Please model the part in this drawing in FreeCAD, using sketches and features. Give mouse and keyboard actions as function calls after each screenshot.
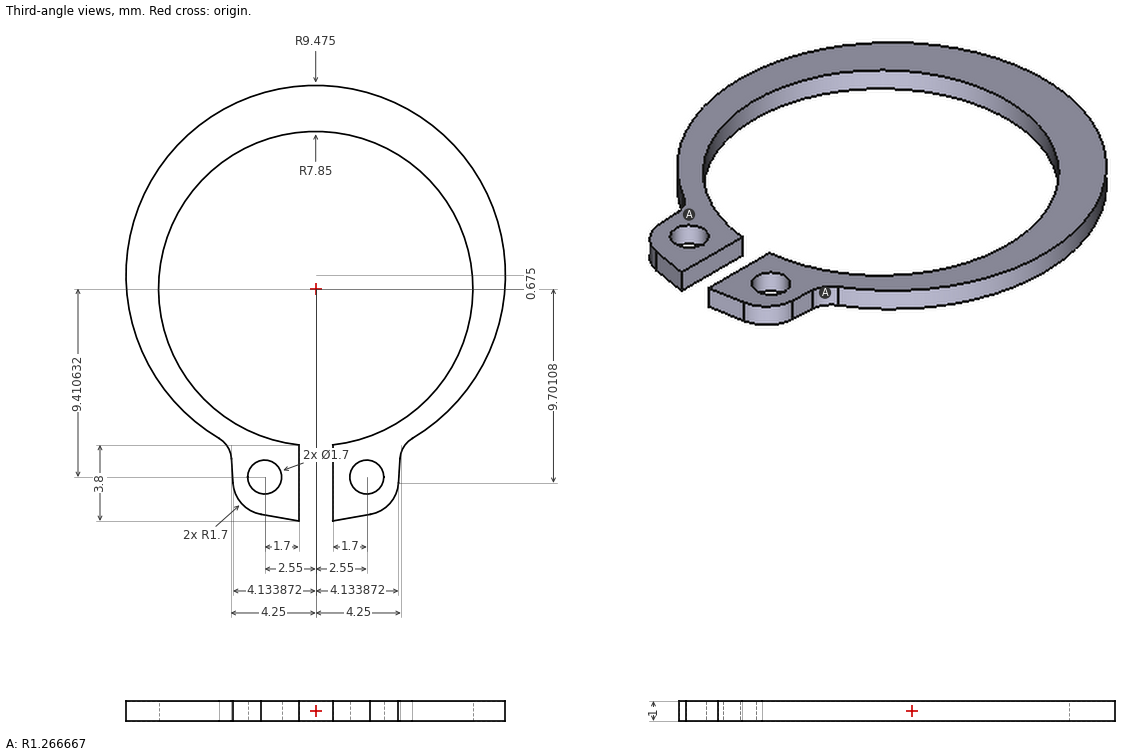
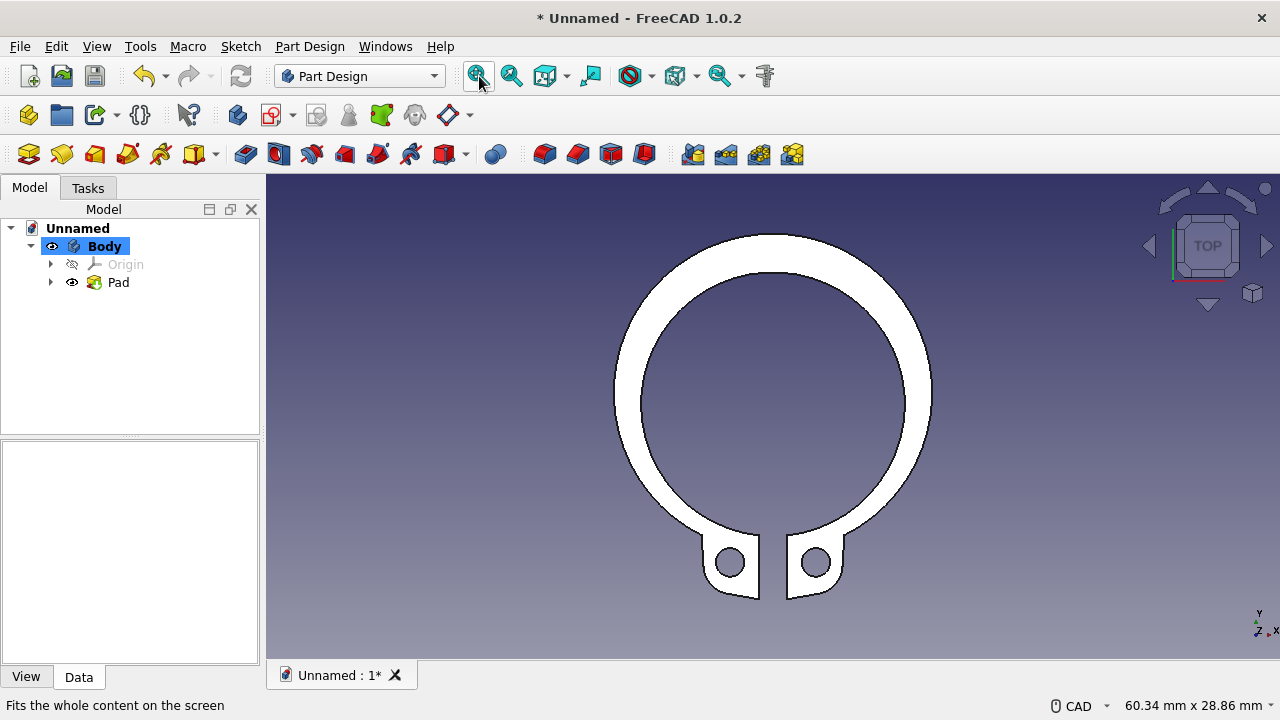
key(1)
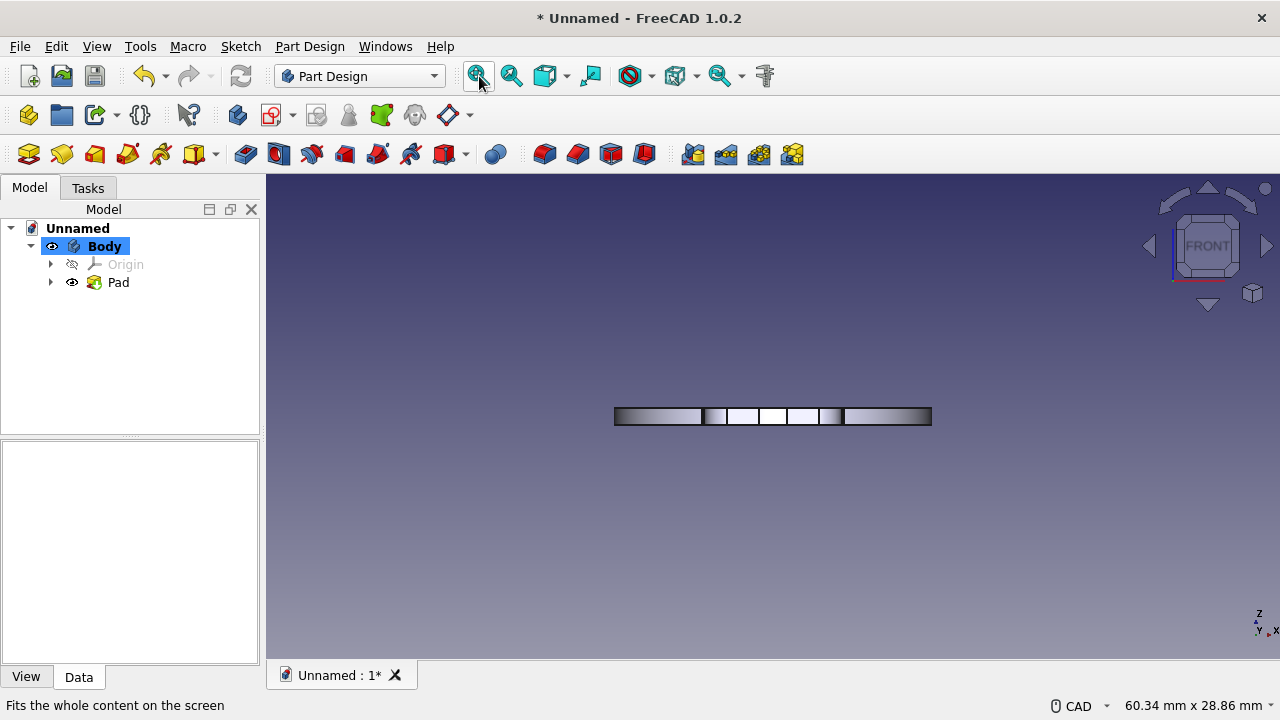
click(479, 76)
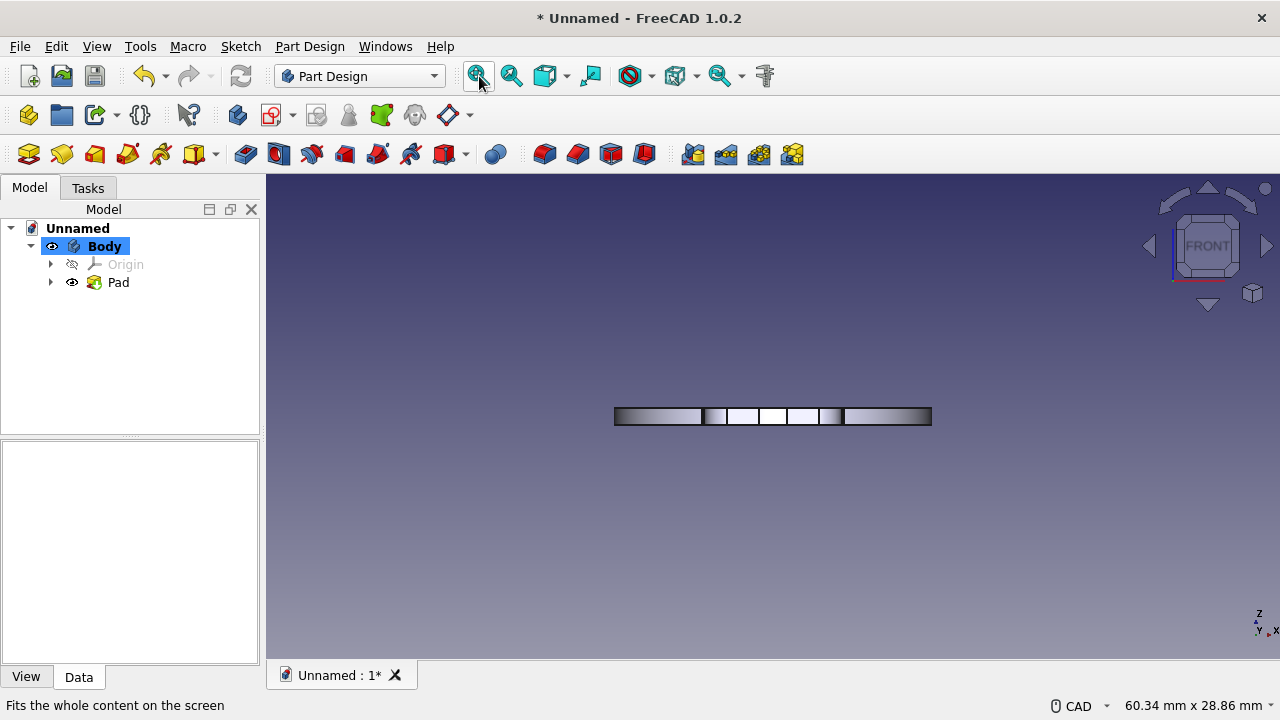
scroll(702, 416, up, 5)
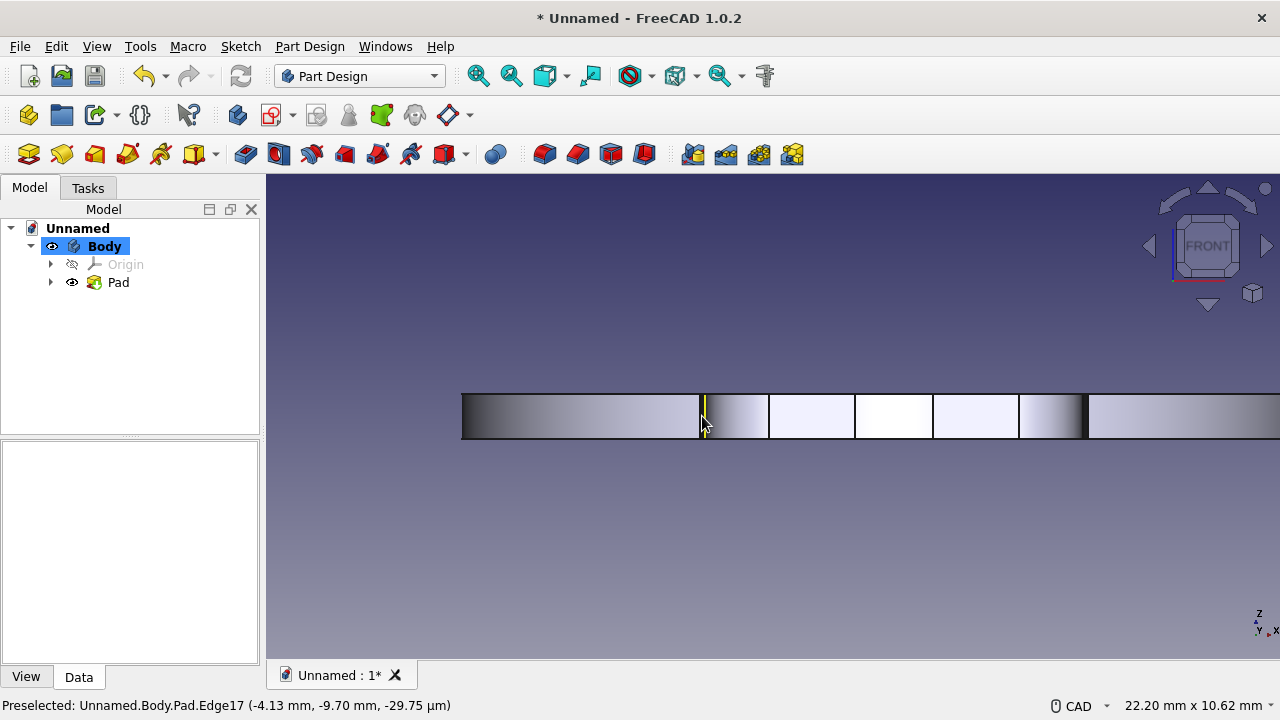
click(479, 76)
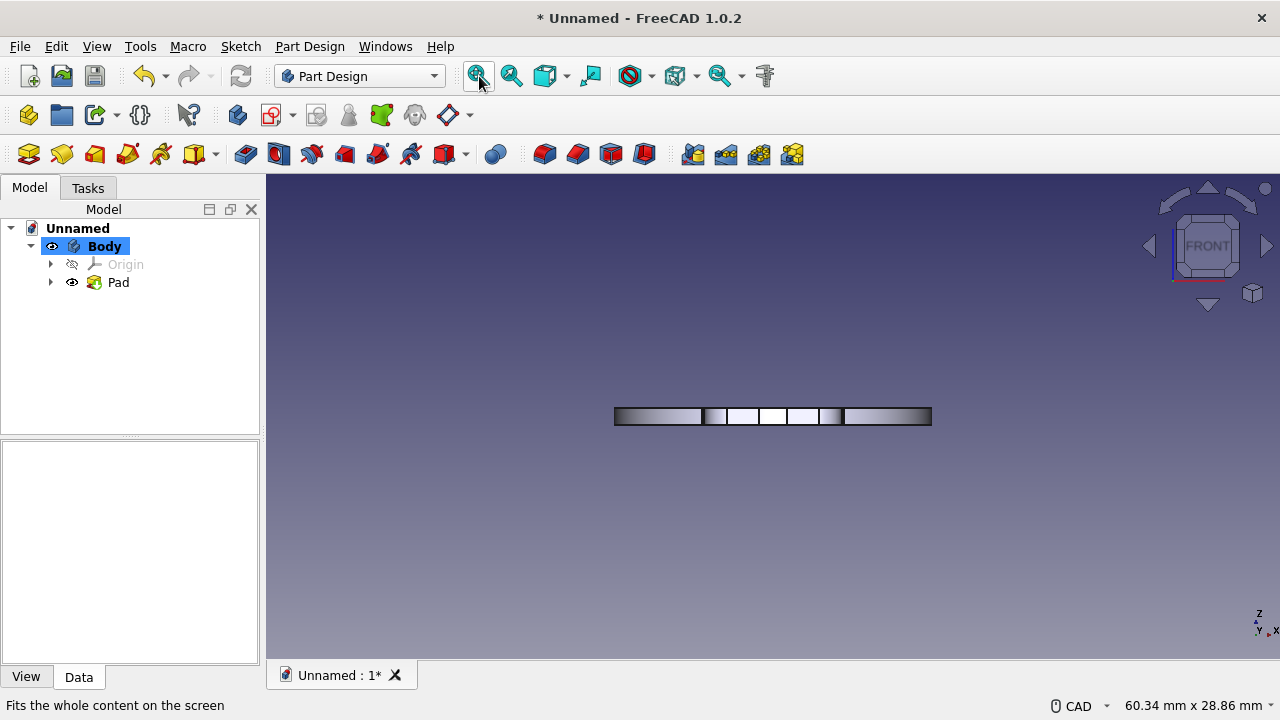
key(3)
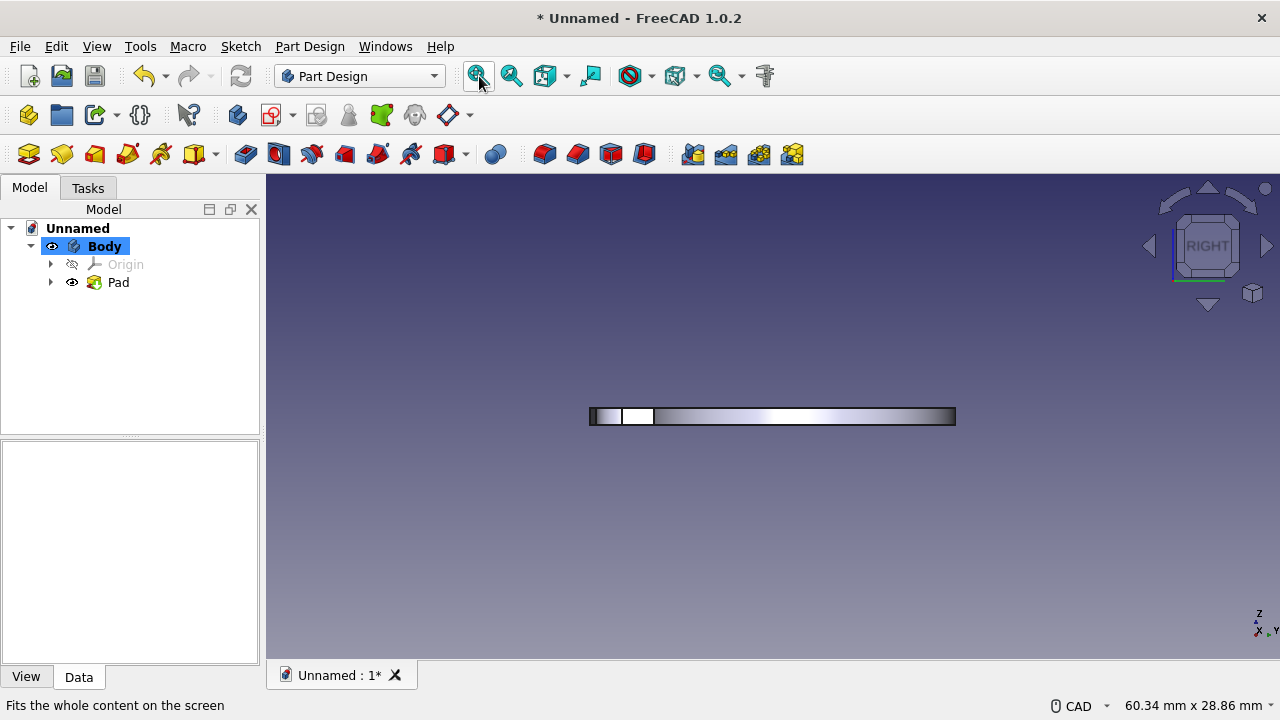
click(479, 76)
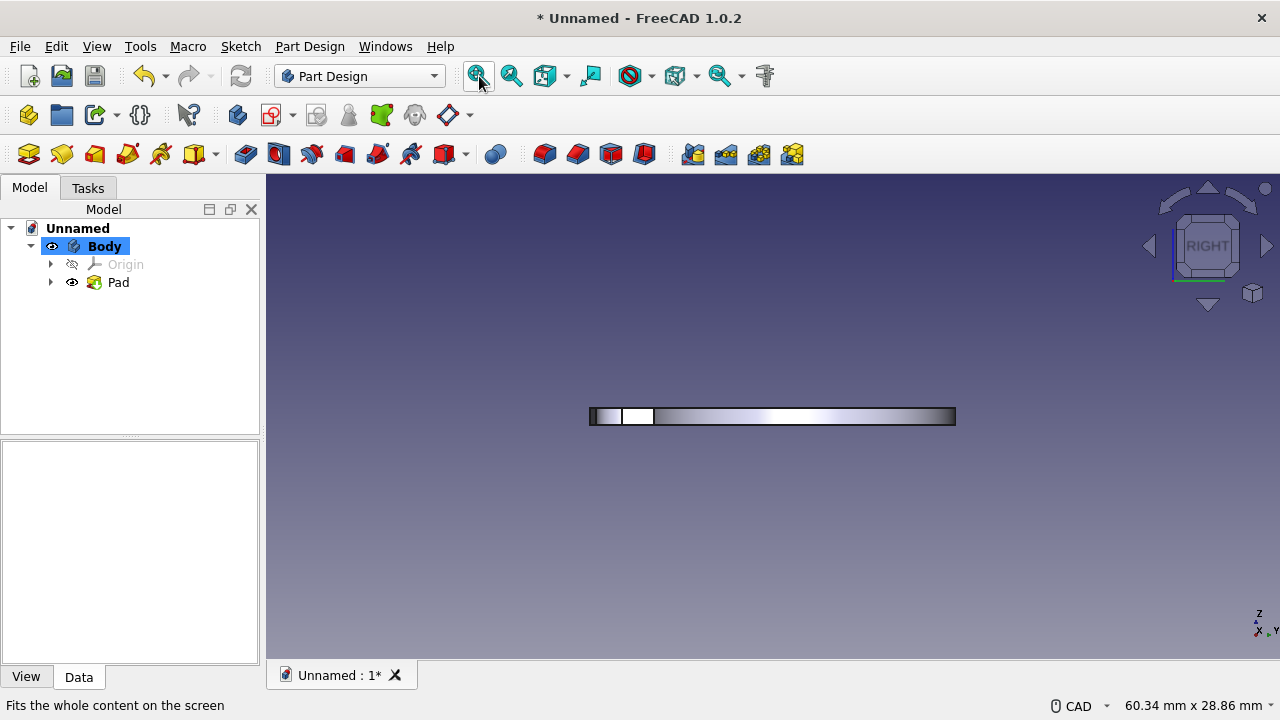
scroll(654, 415, up, 5)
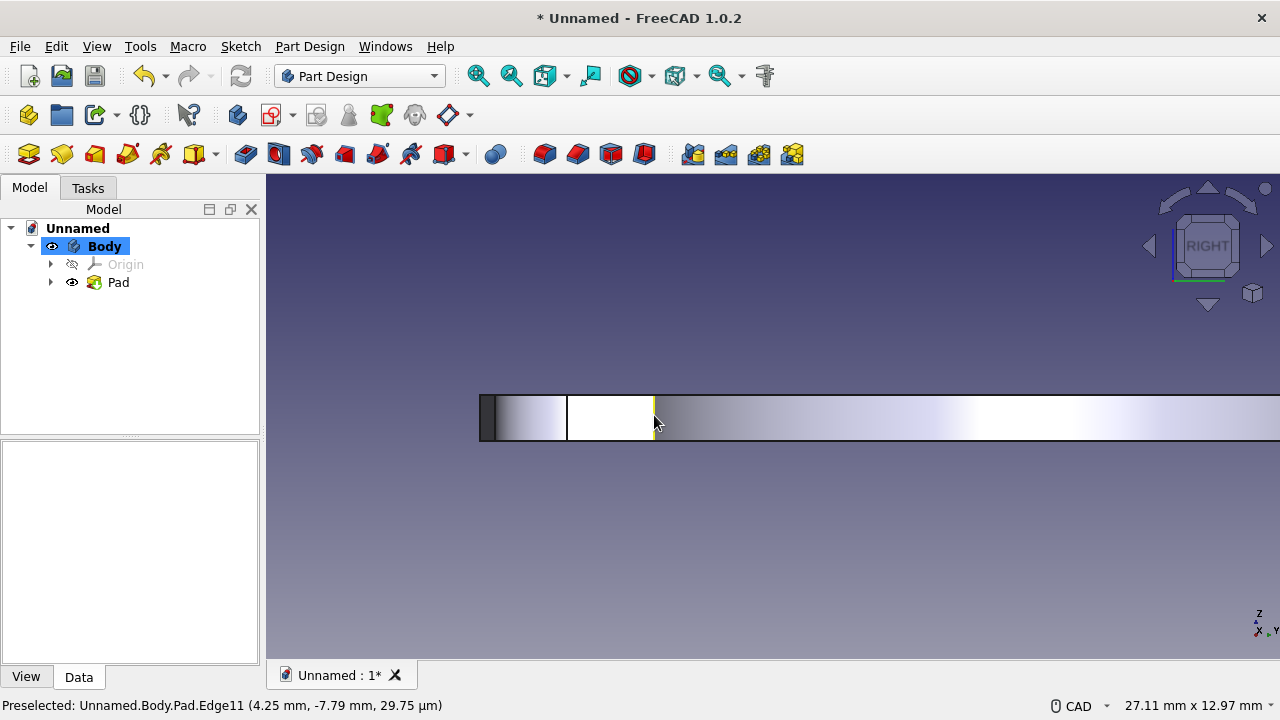
click(479, 76)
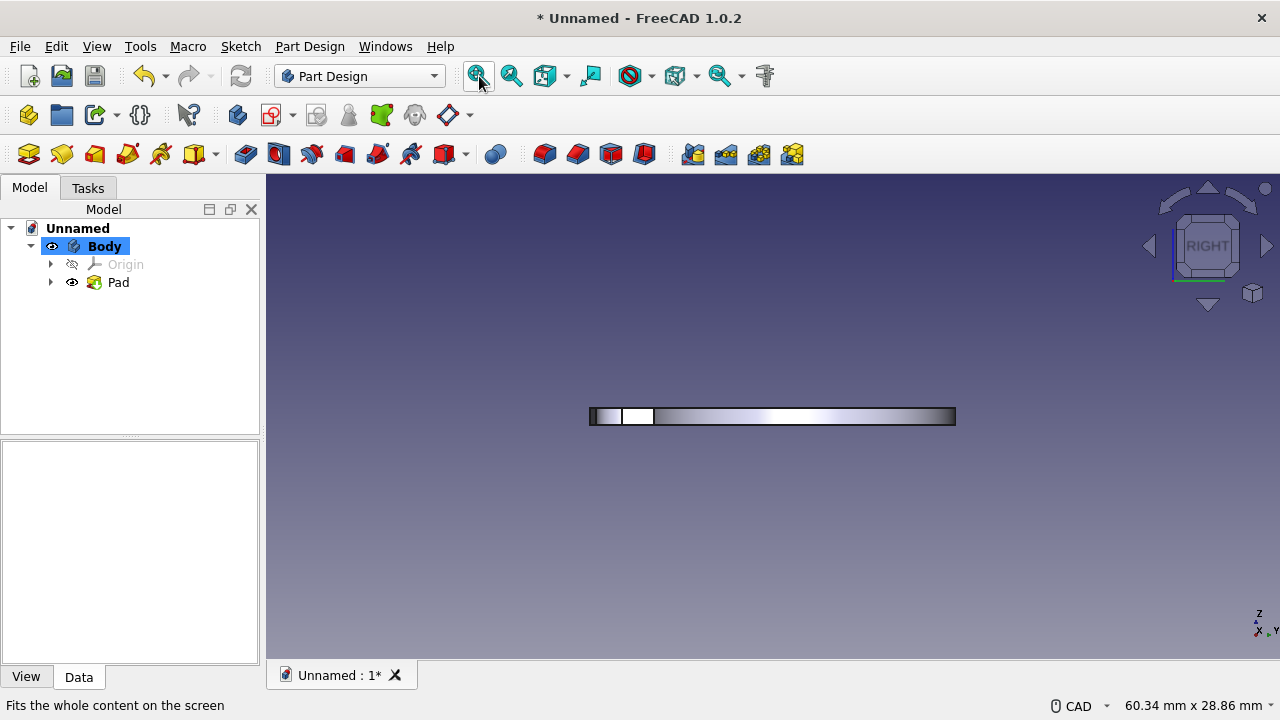
key(5)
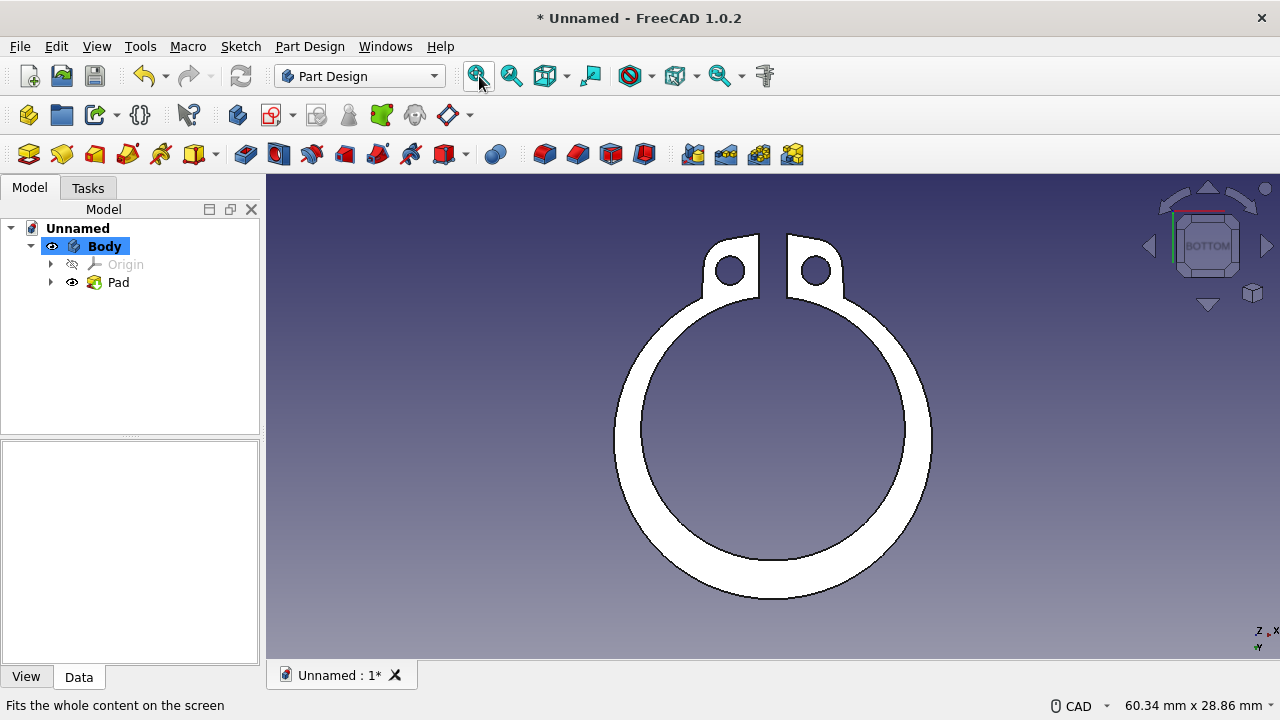
scroll(702, 297, up, 5)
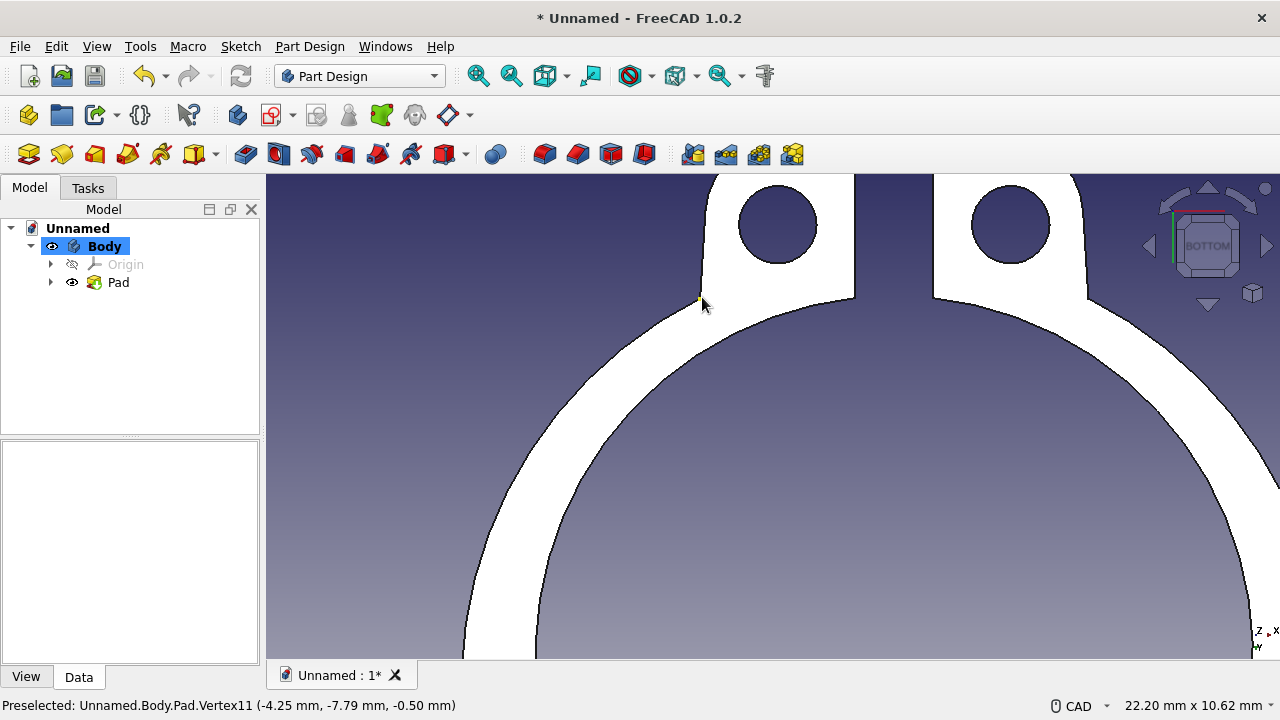
click(479, 76)